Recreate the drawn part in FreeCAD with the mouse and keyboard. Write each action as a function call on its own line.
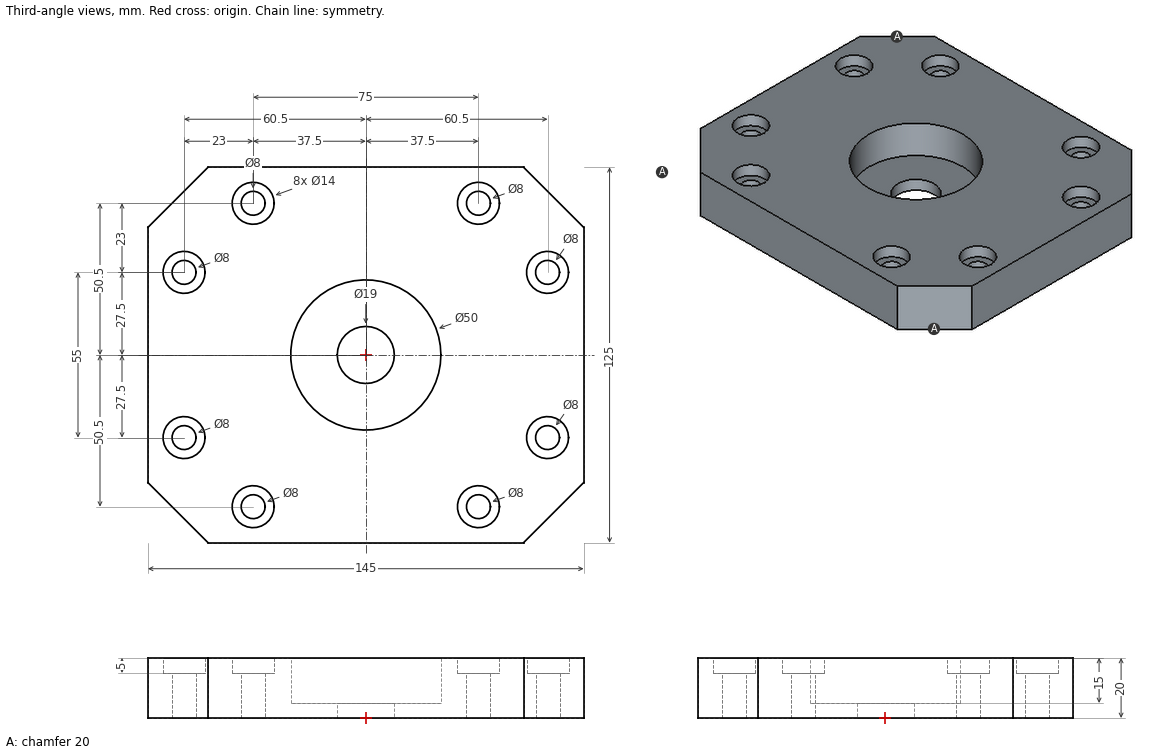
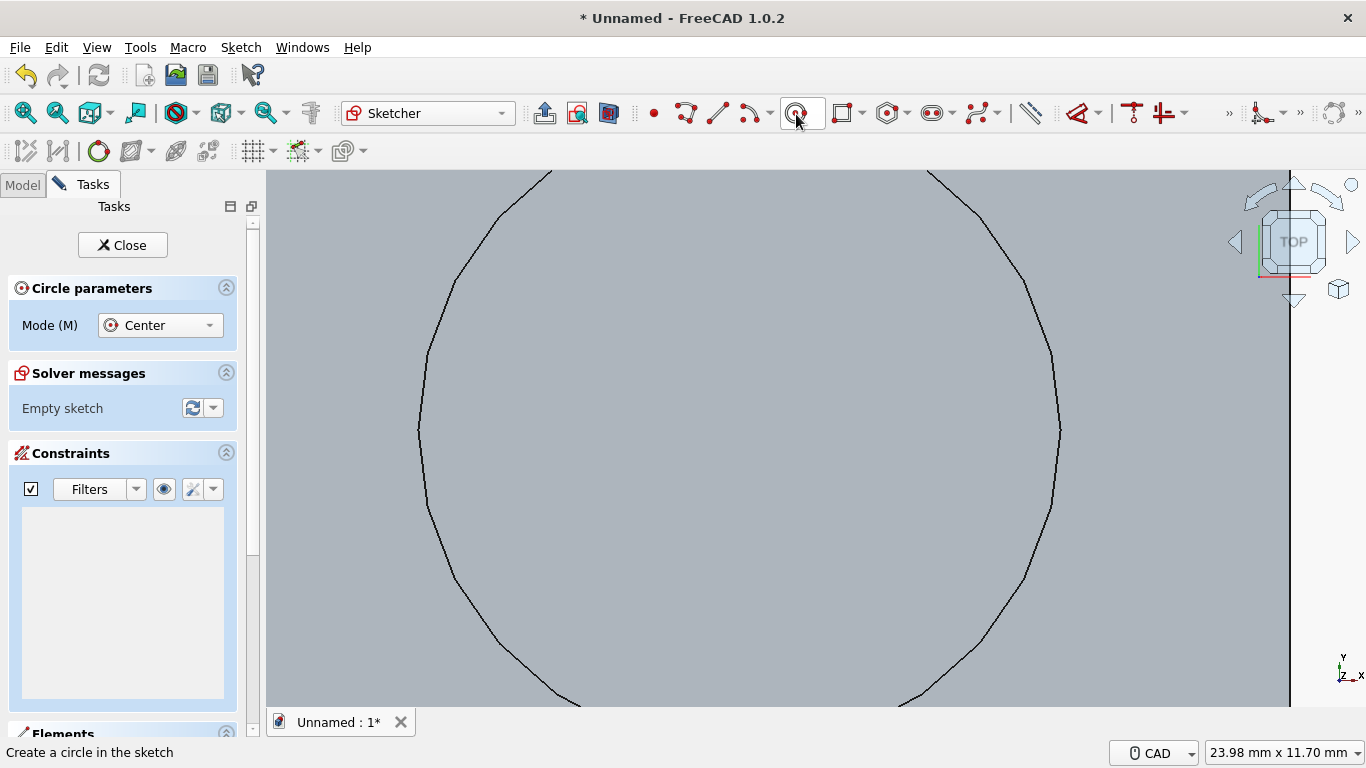
click(739, 430)
click(869, 300)
key(Escape)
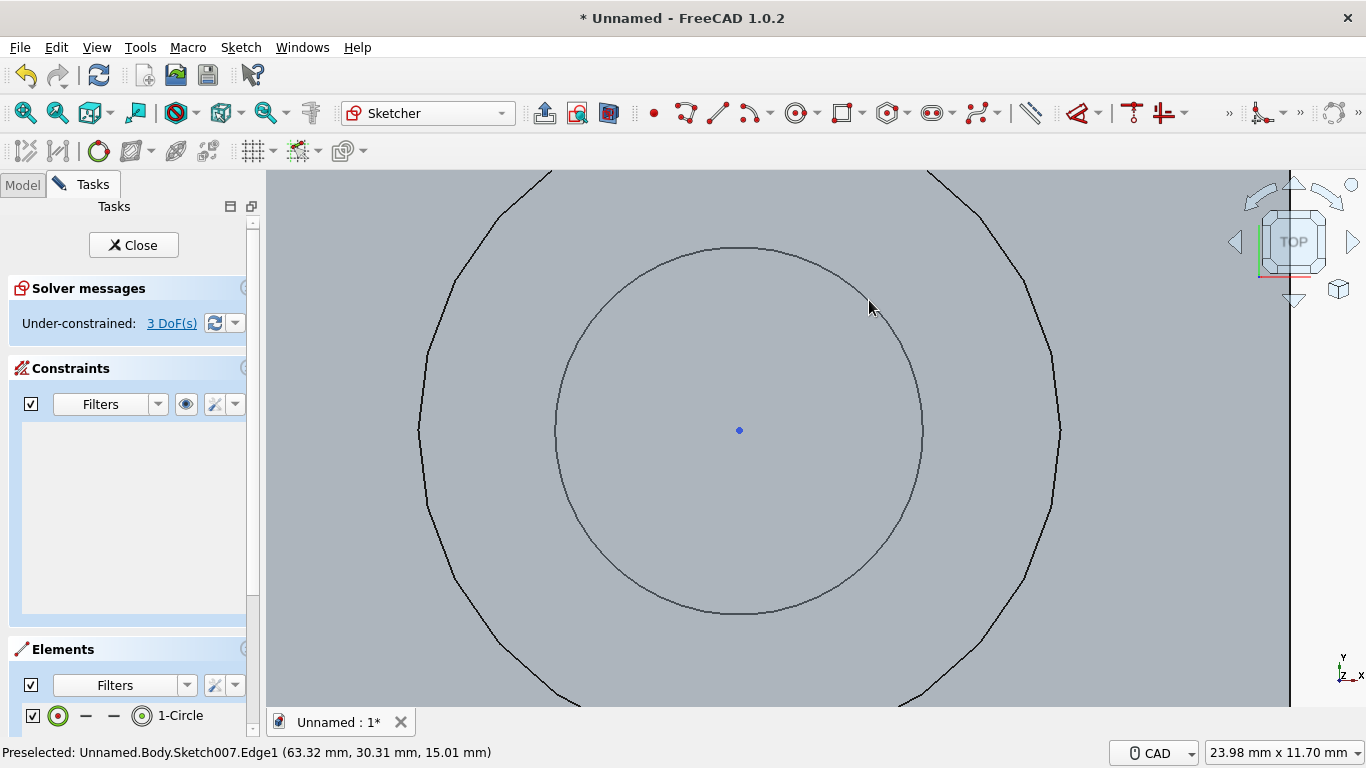
click(1078, 114)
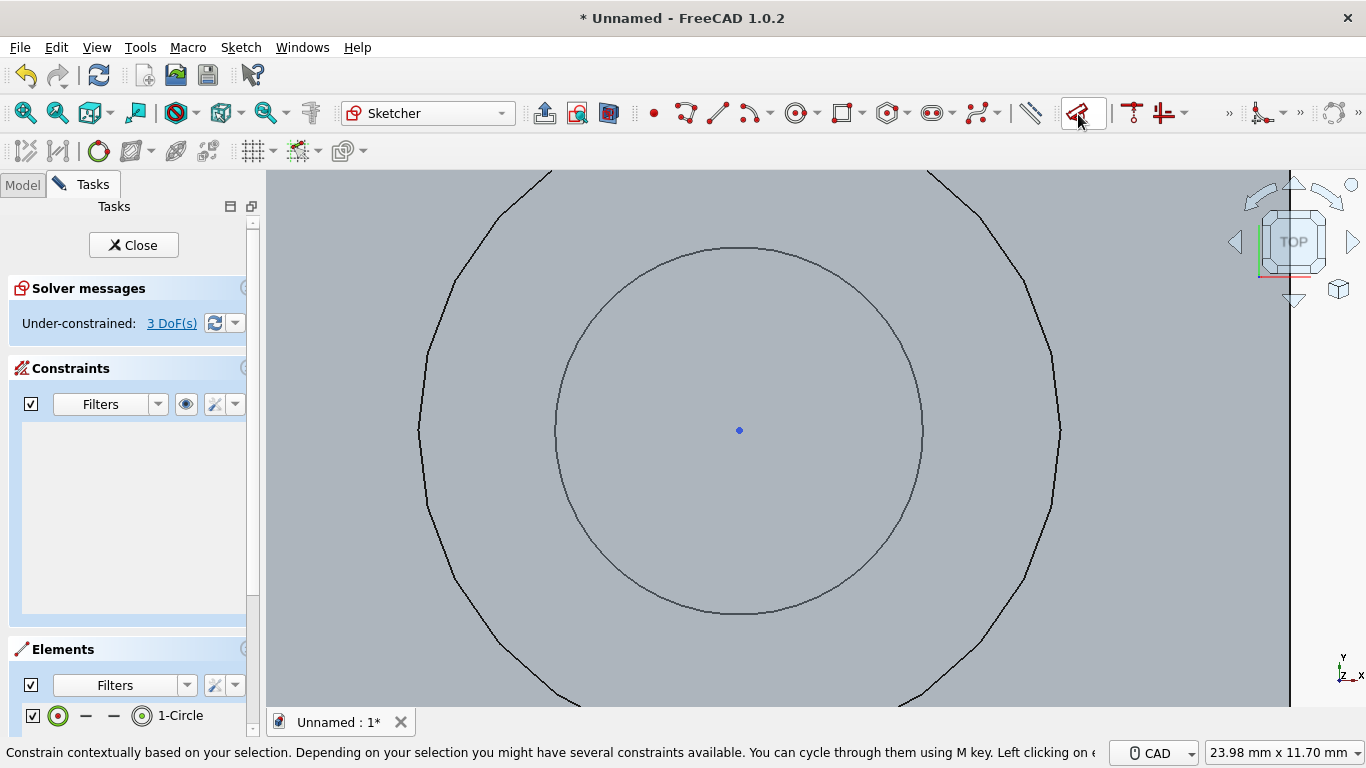
click(869, 301)
click(892, 278)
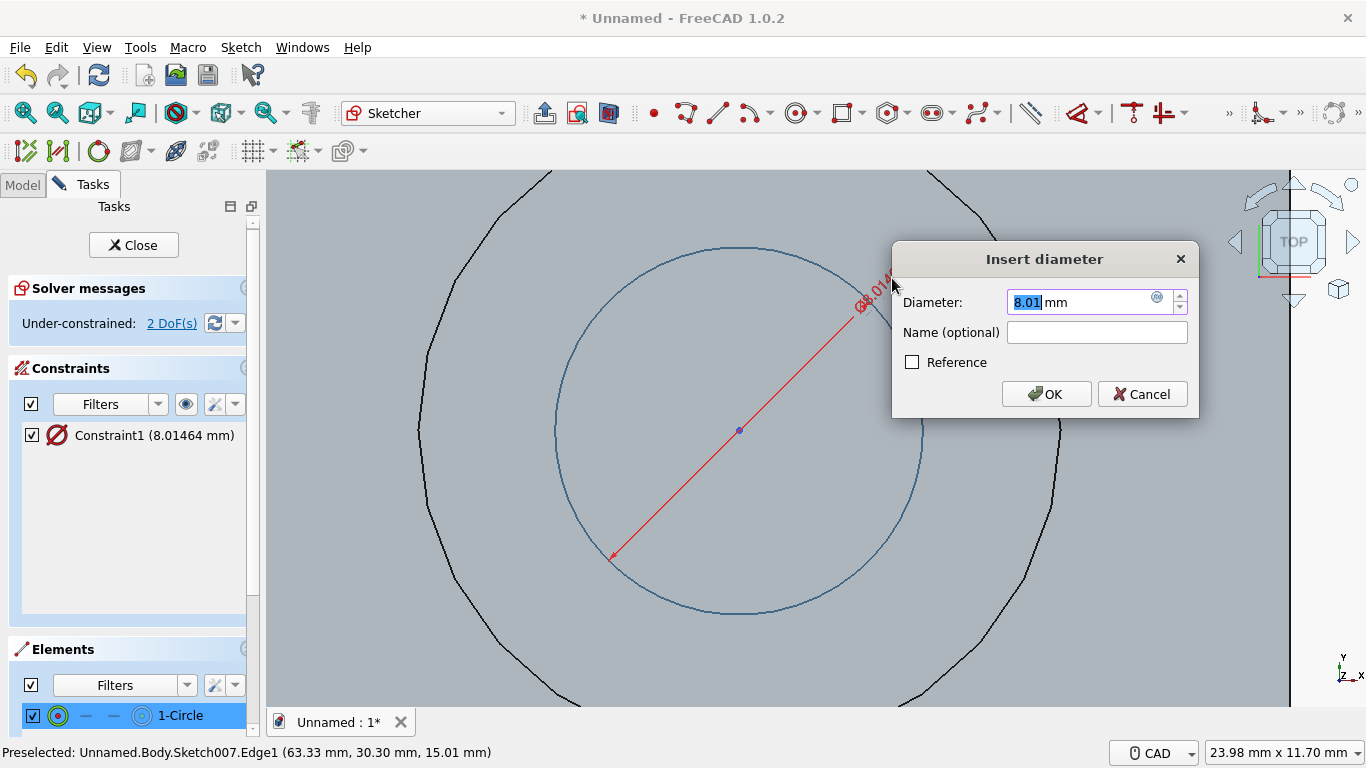
text(8)
key(Return)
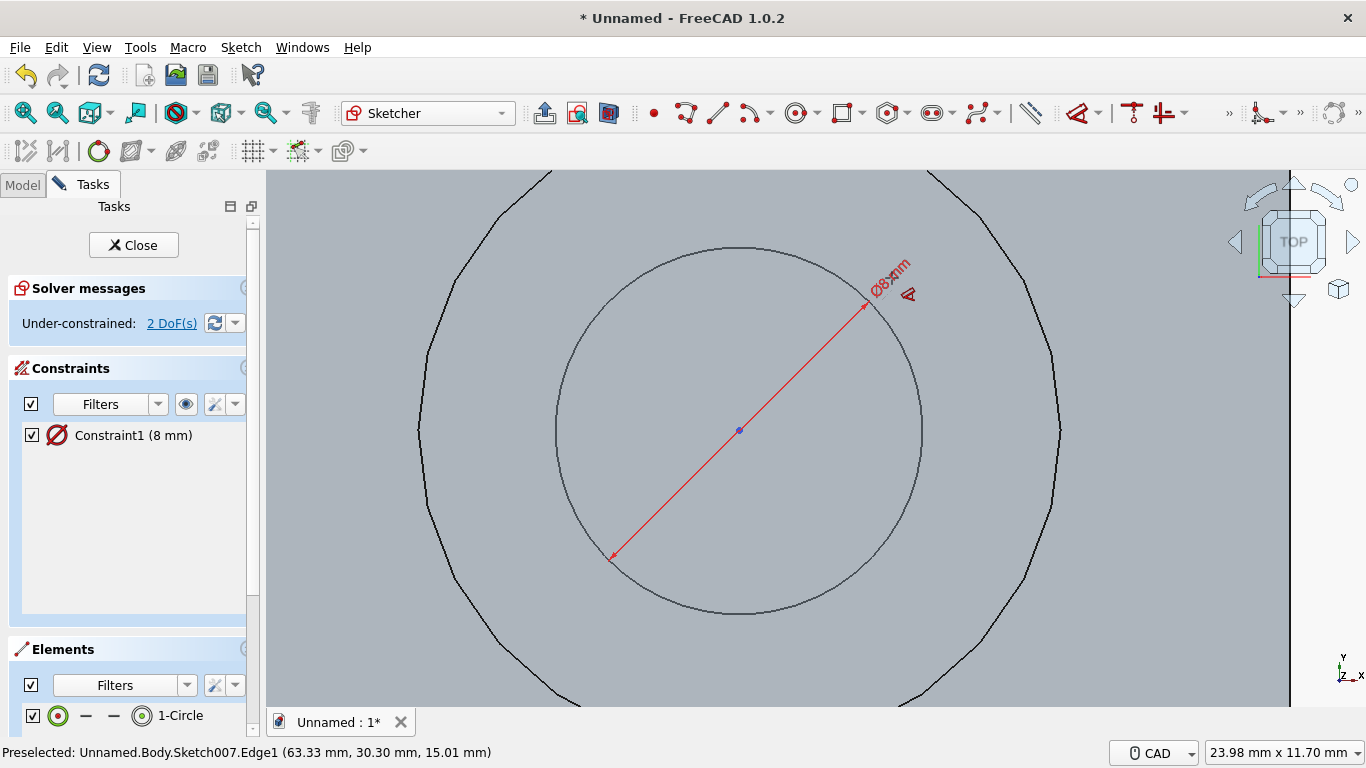
click(739, 431)
click(516, 397)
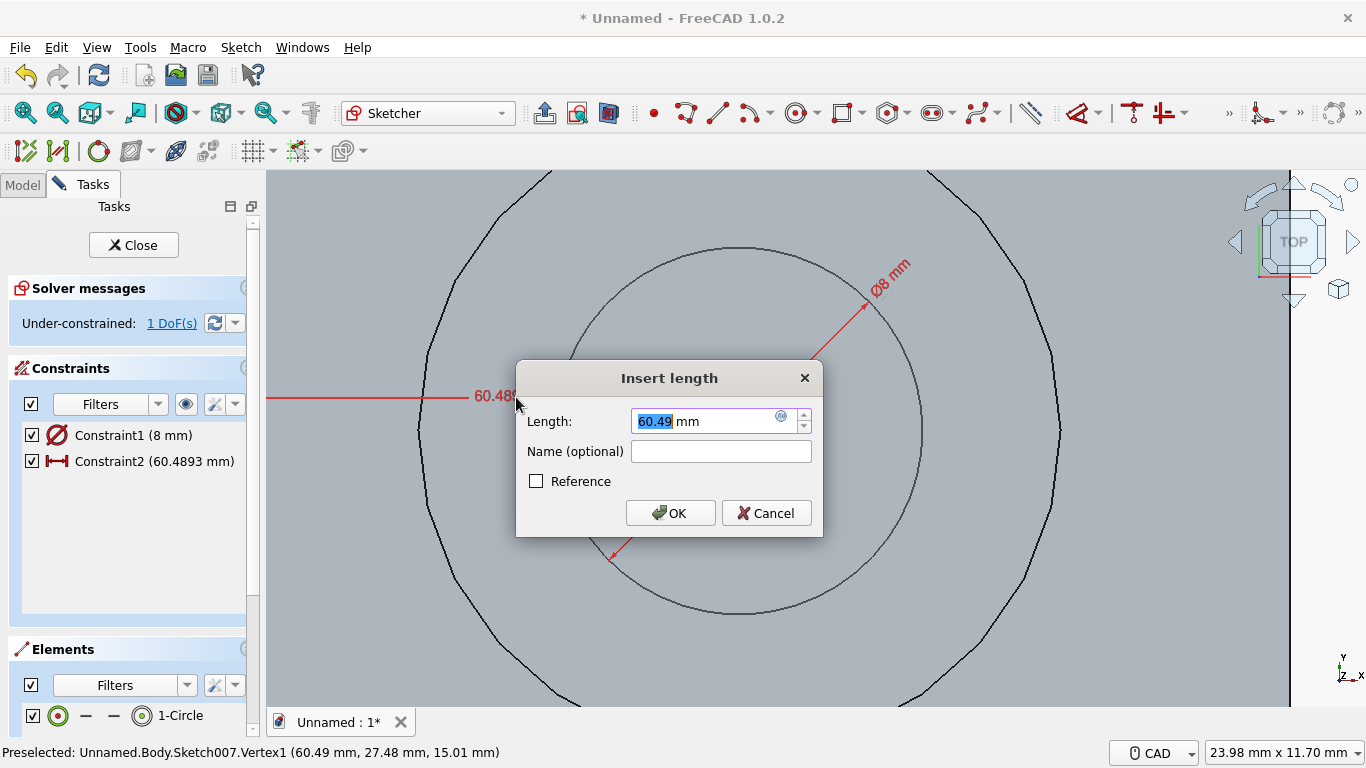
text(60.5)
key(Return)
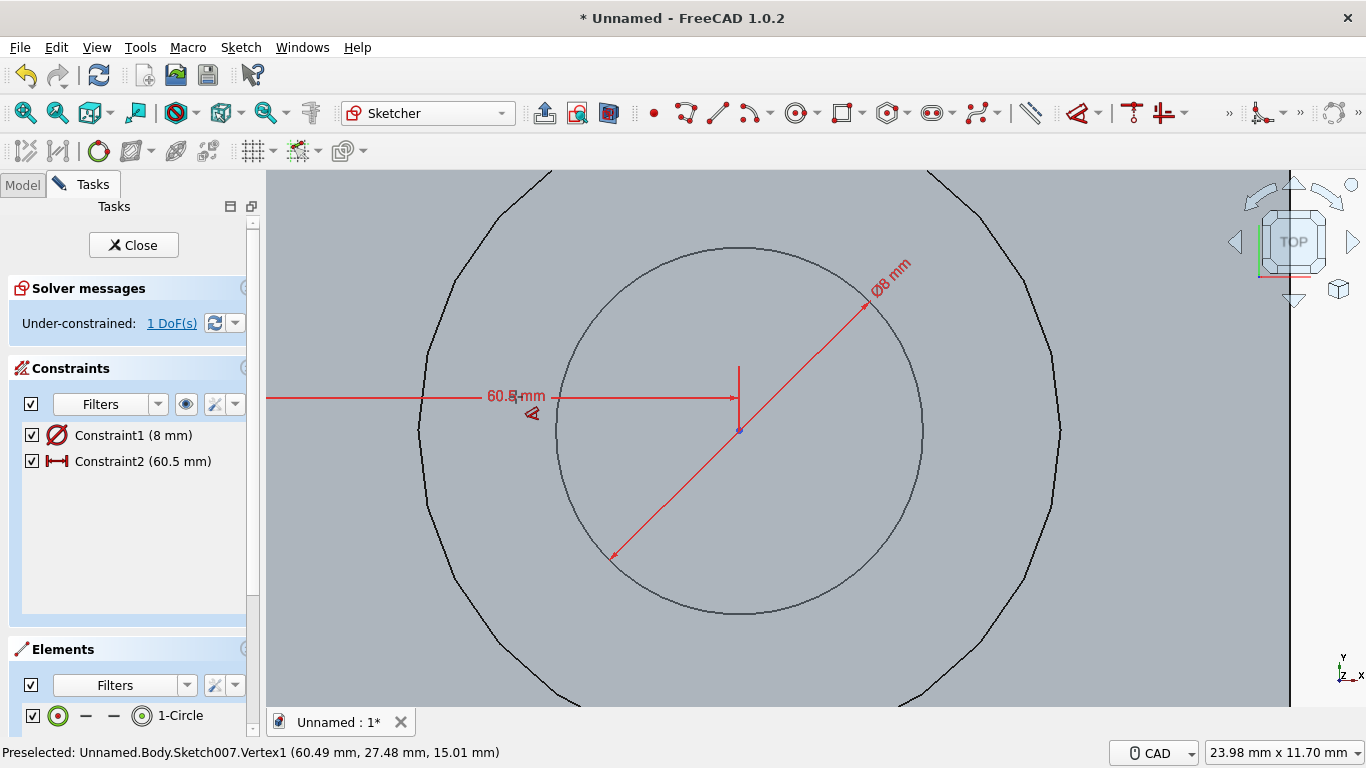
click(739, 431)
click(773, 555)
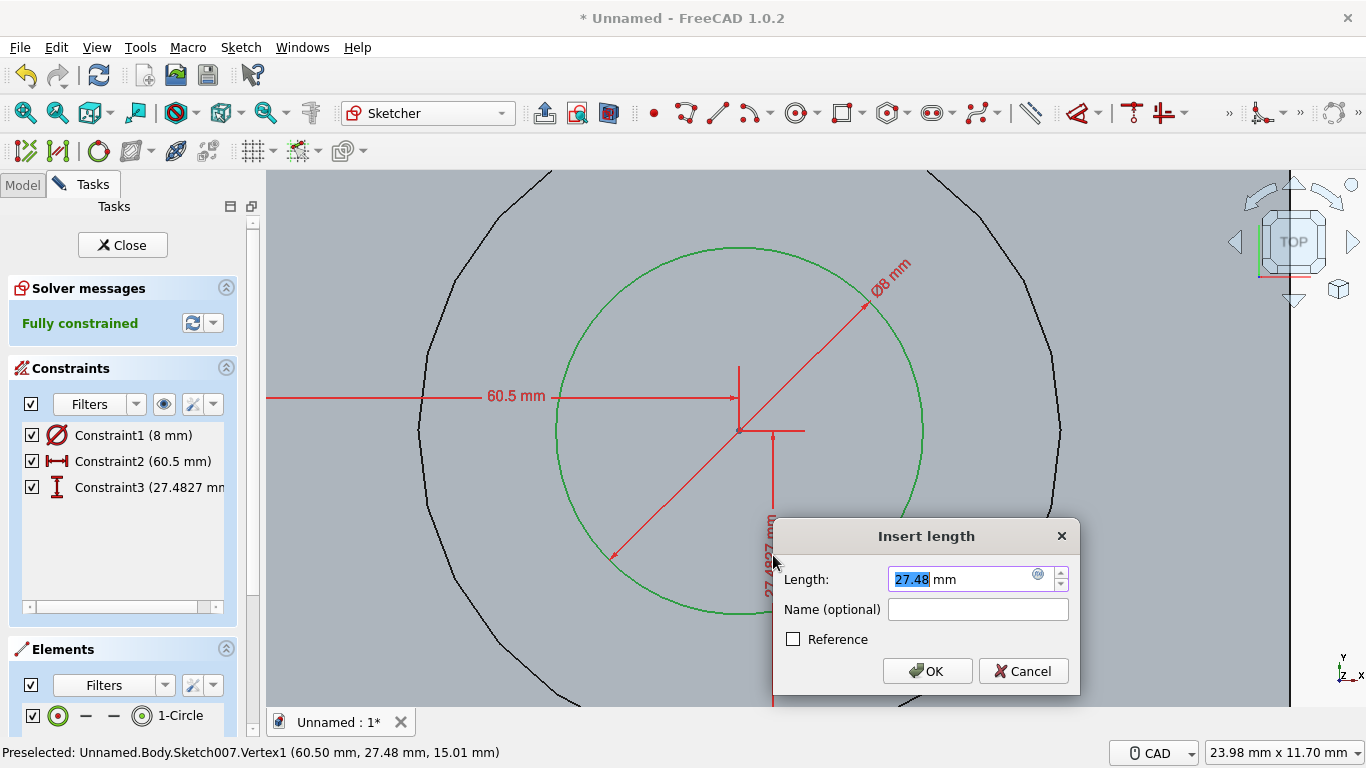
text(27.5)
key(Return)
key(Escape)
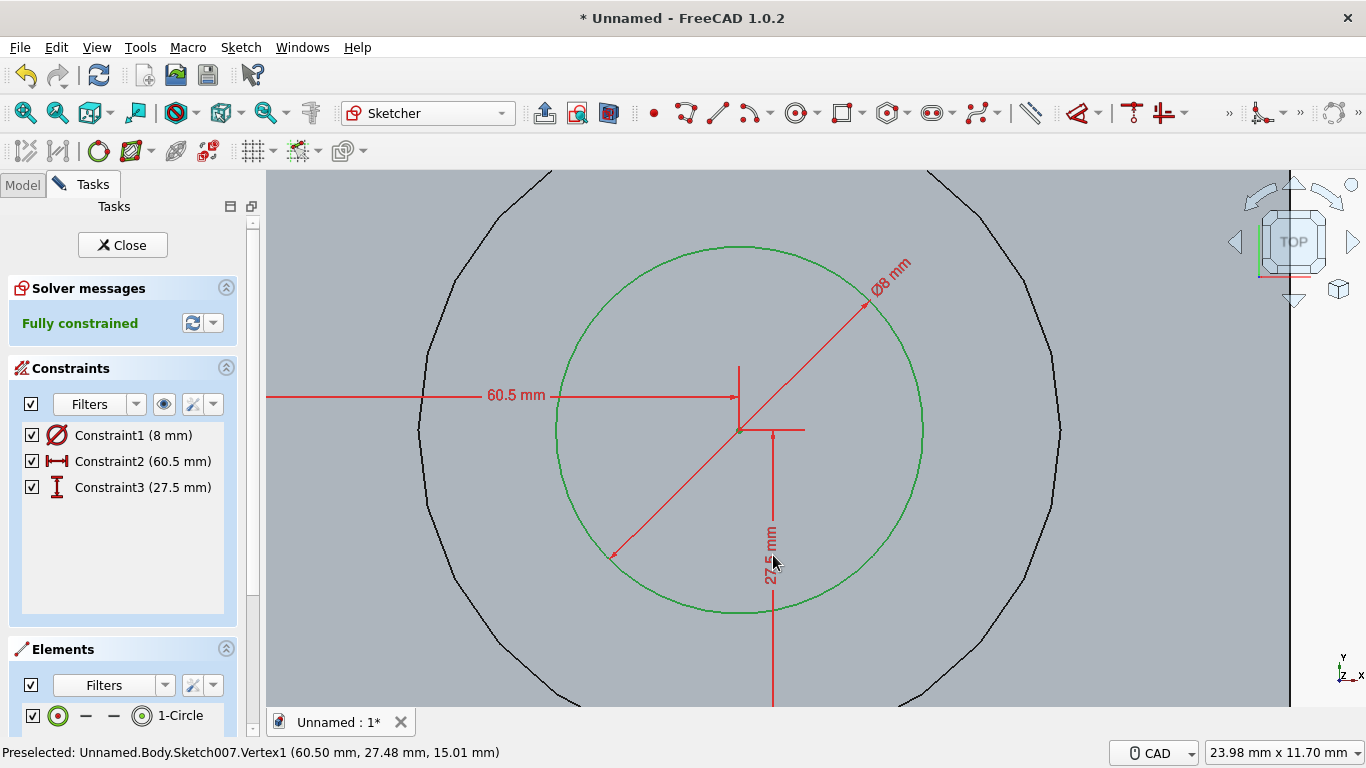
click(123, 245)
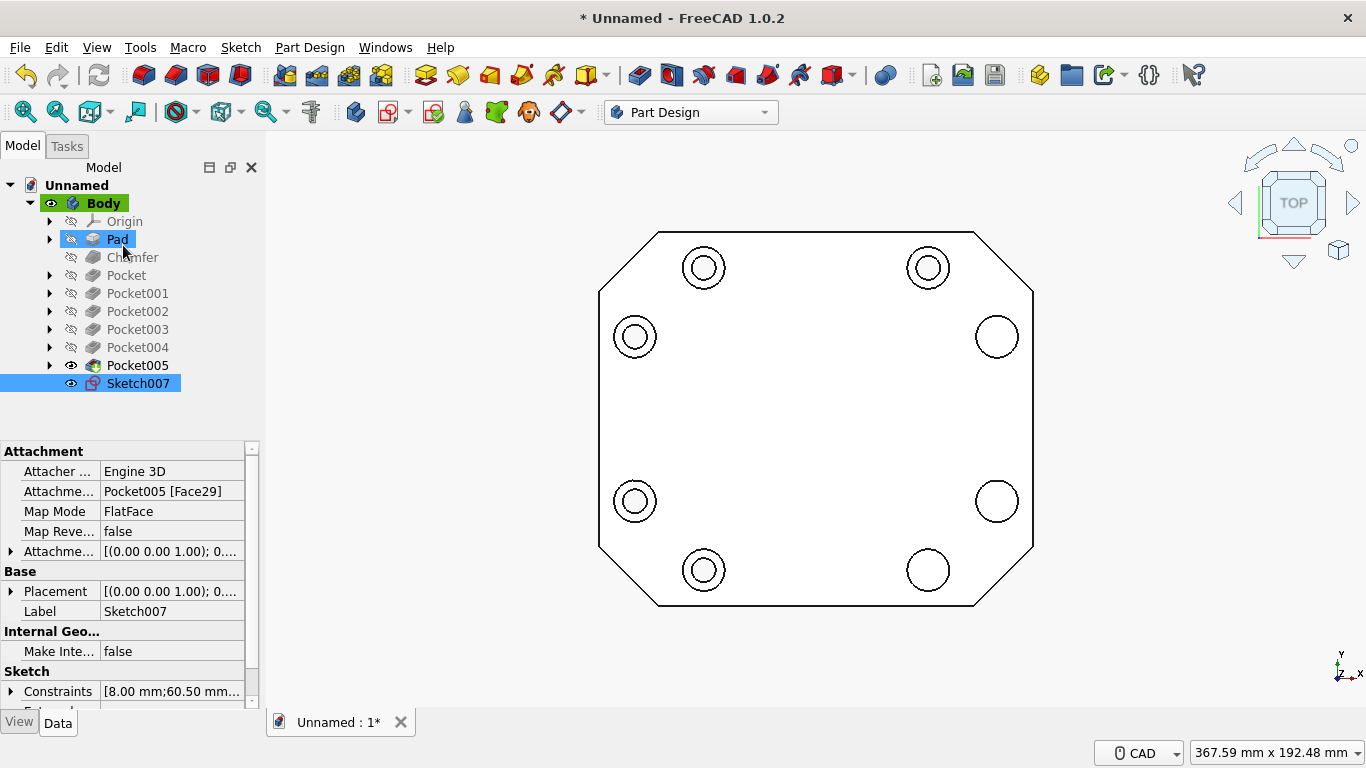
click(640, 76)